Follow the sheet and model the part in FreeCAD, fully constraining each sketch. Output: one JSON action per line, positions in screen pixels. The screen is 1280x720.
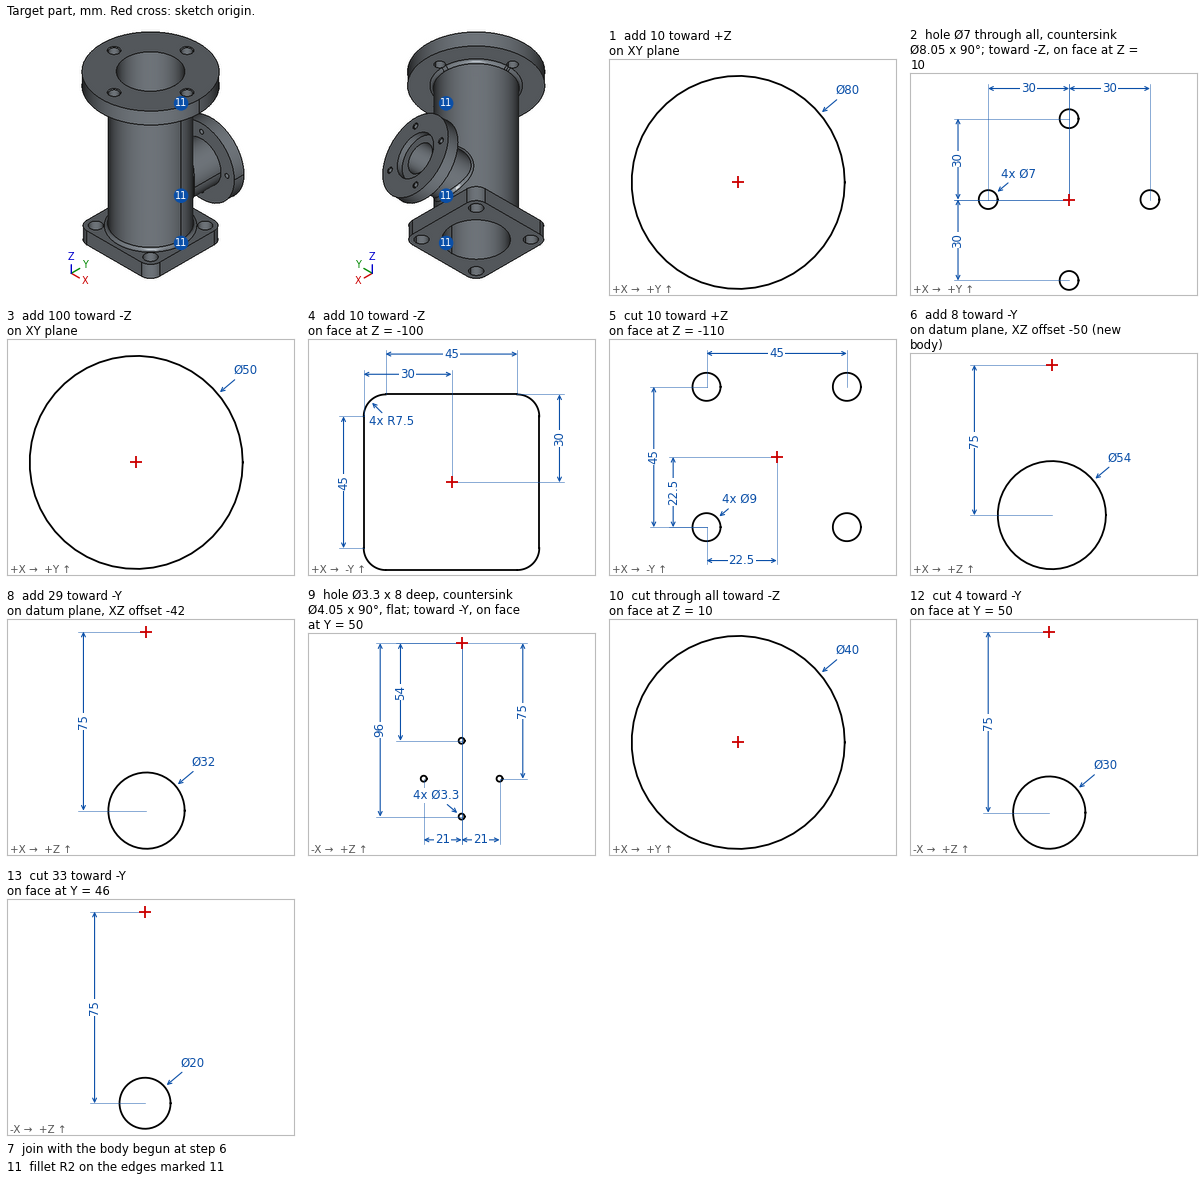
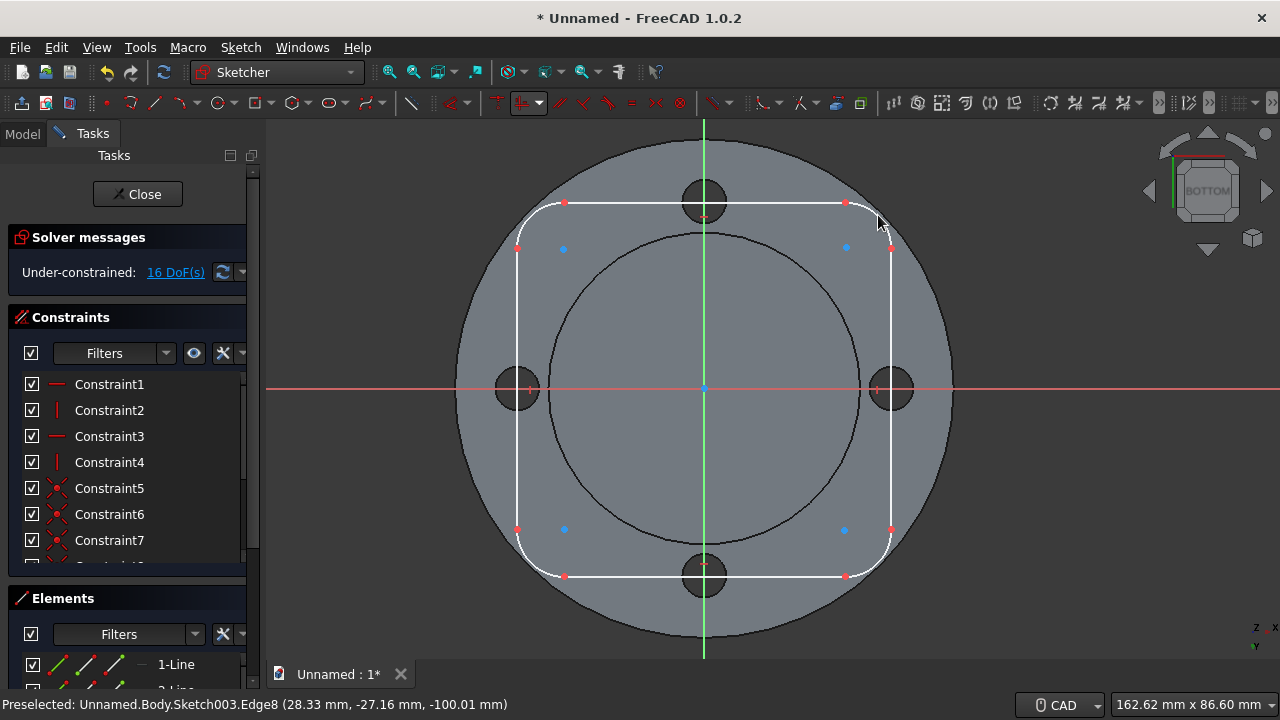
{"action": "left_click", "coordinate": [761, 203]}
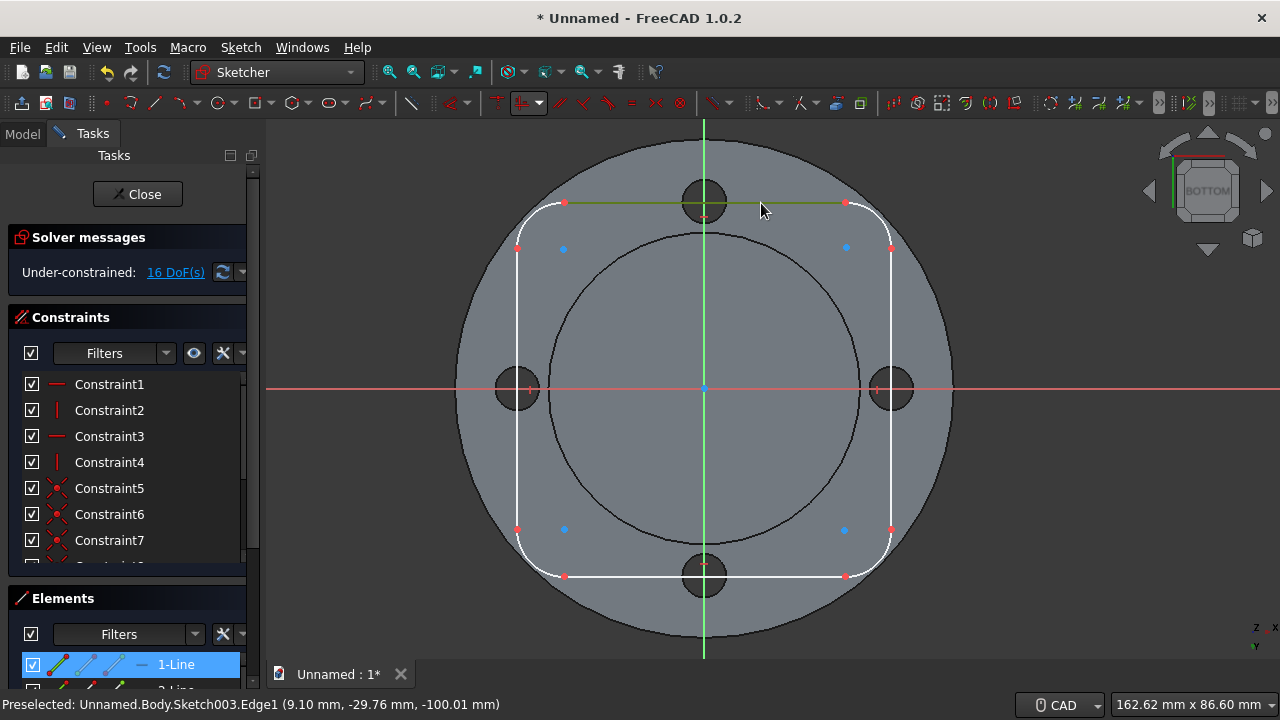
{"action": "left_click", "coordinate": [543, 208]}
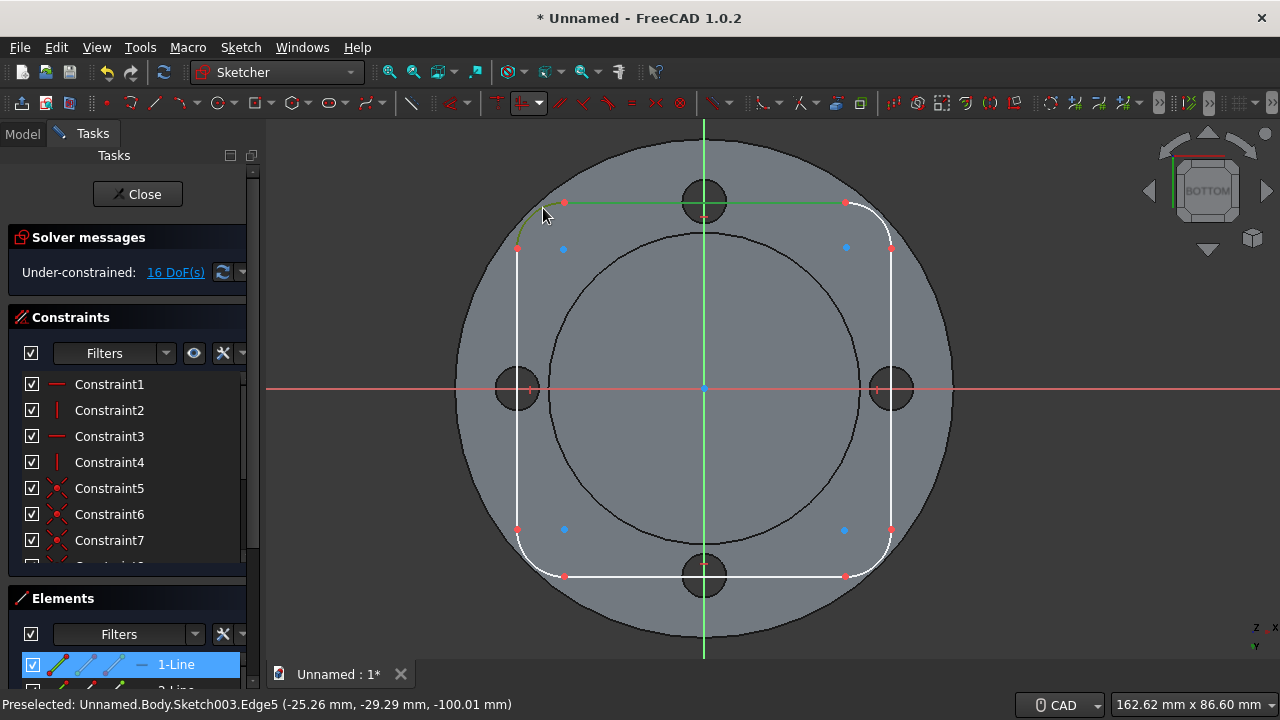
{"action": "left_click", "coordinate": [608, 104]}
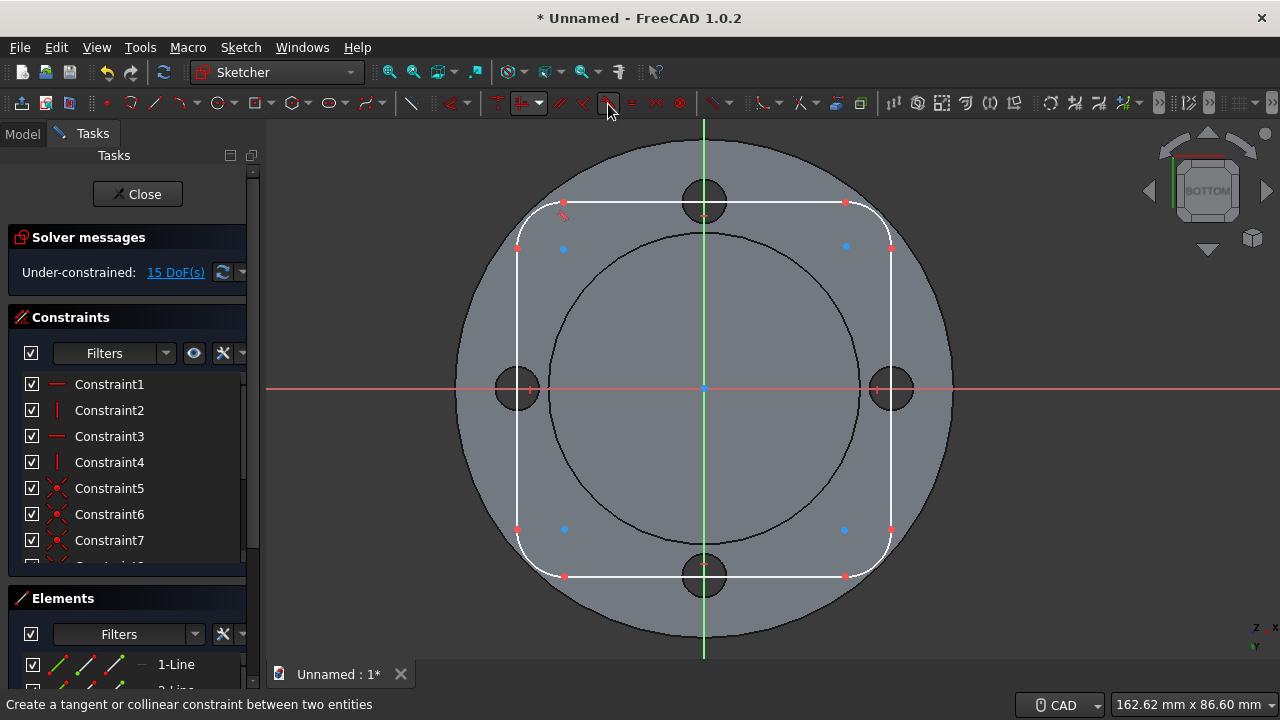
{"action": "left_click", "coordinate": [761, 202]}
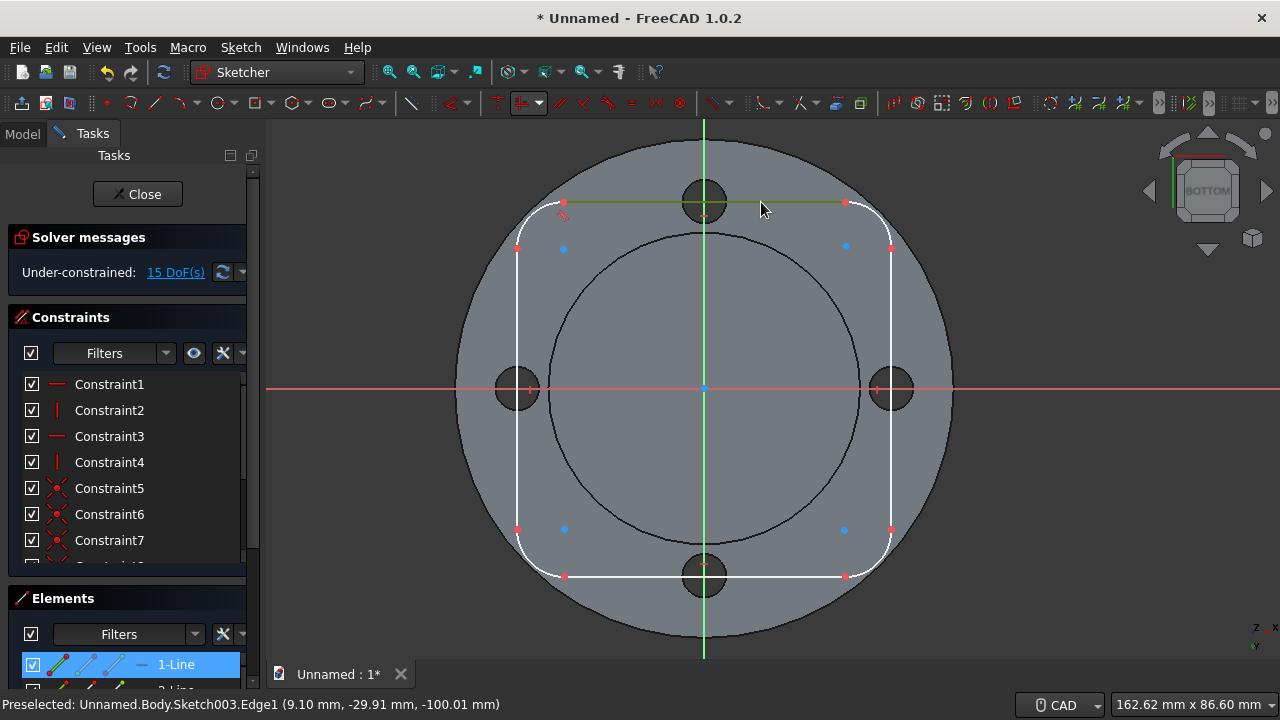
{"action": "left_click", "coordinate": [887, 228]}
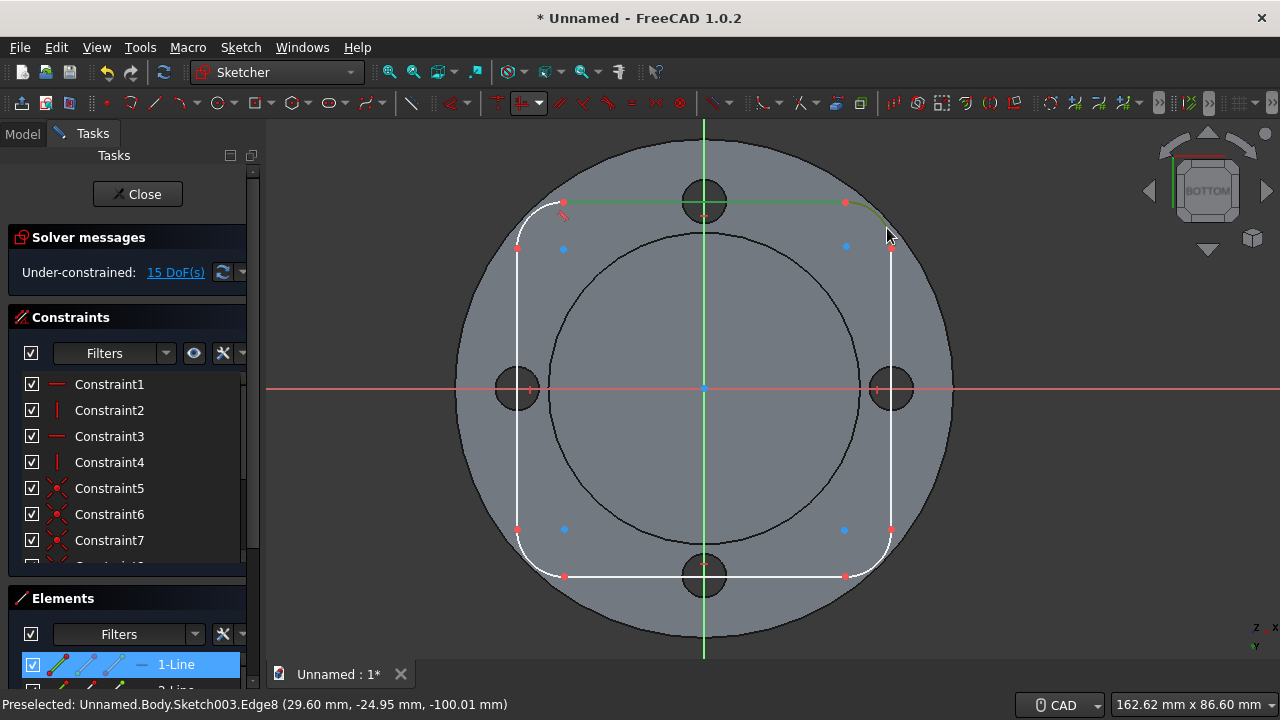
{"action": "left_click", "coordinate": [608, 104]}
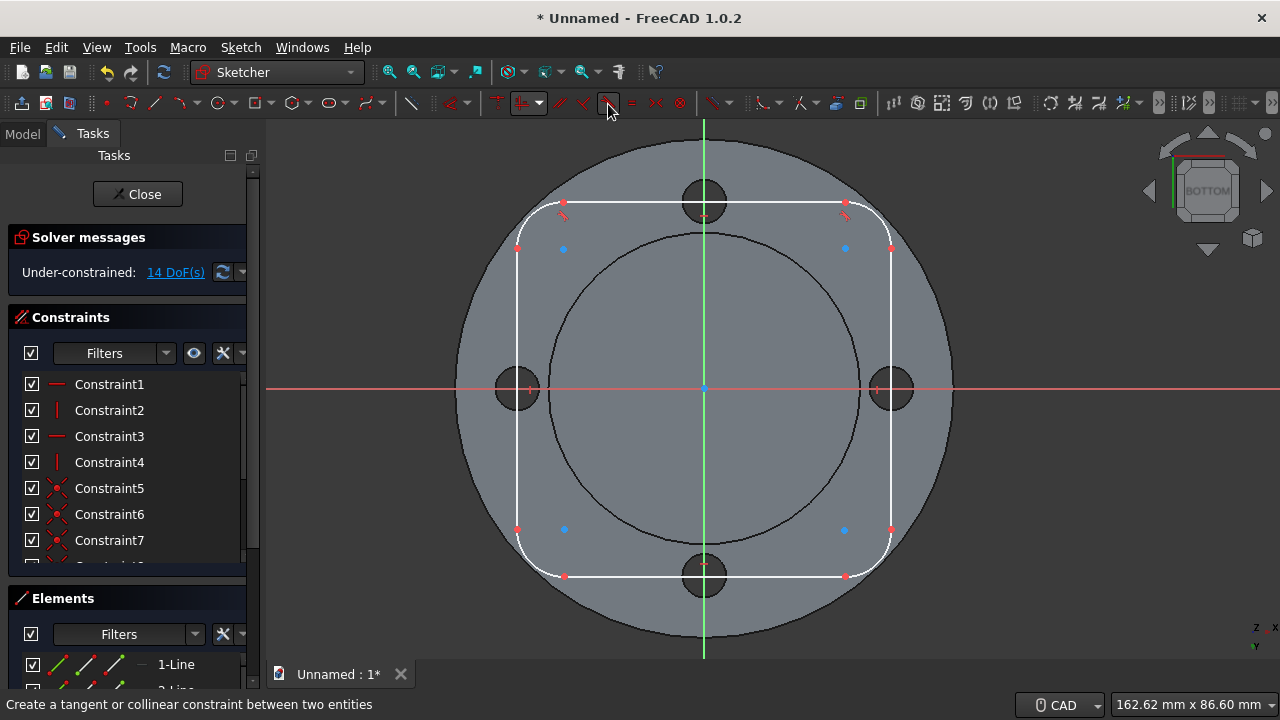
{"action": "left_click", "coordinate": [517, 333]}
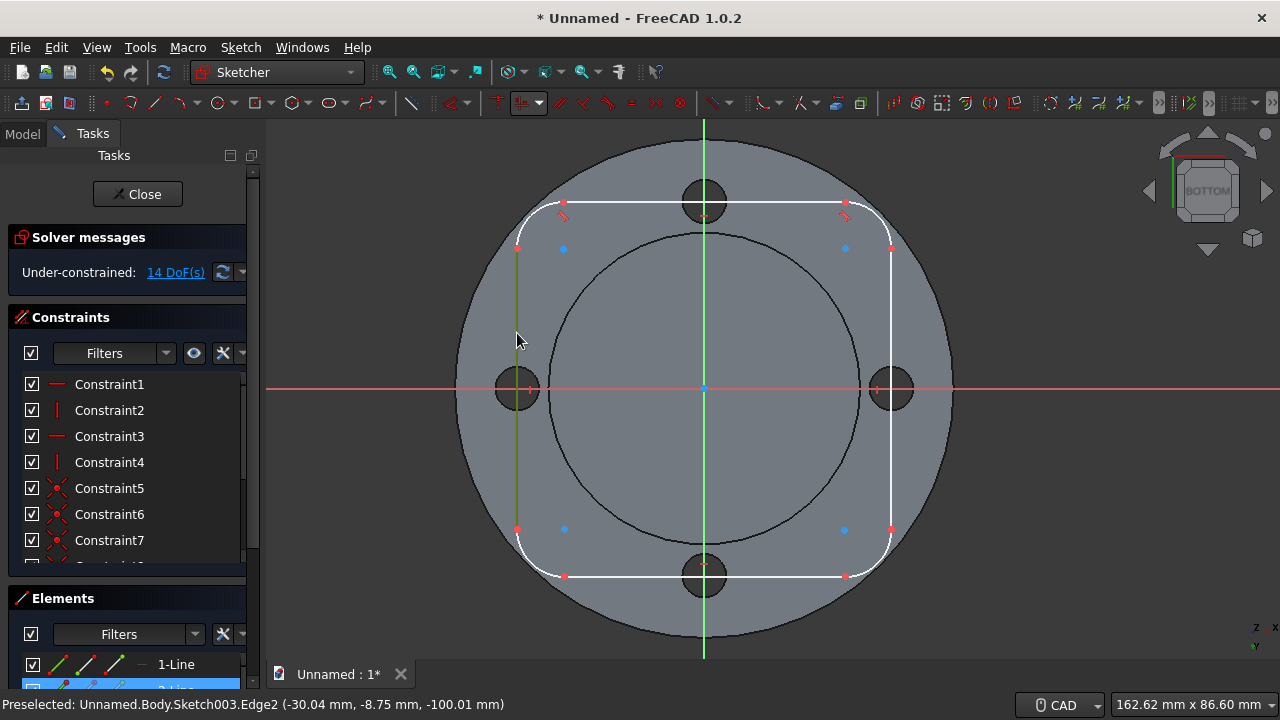
{"action": "left_click", "coordinate": [543, 207]}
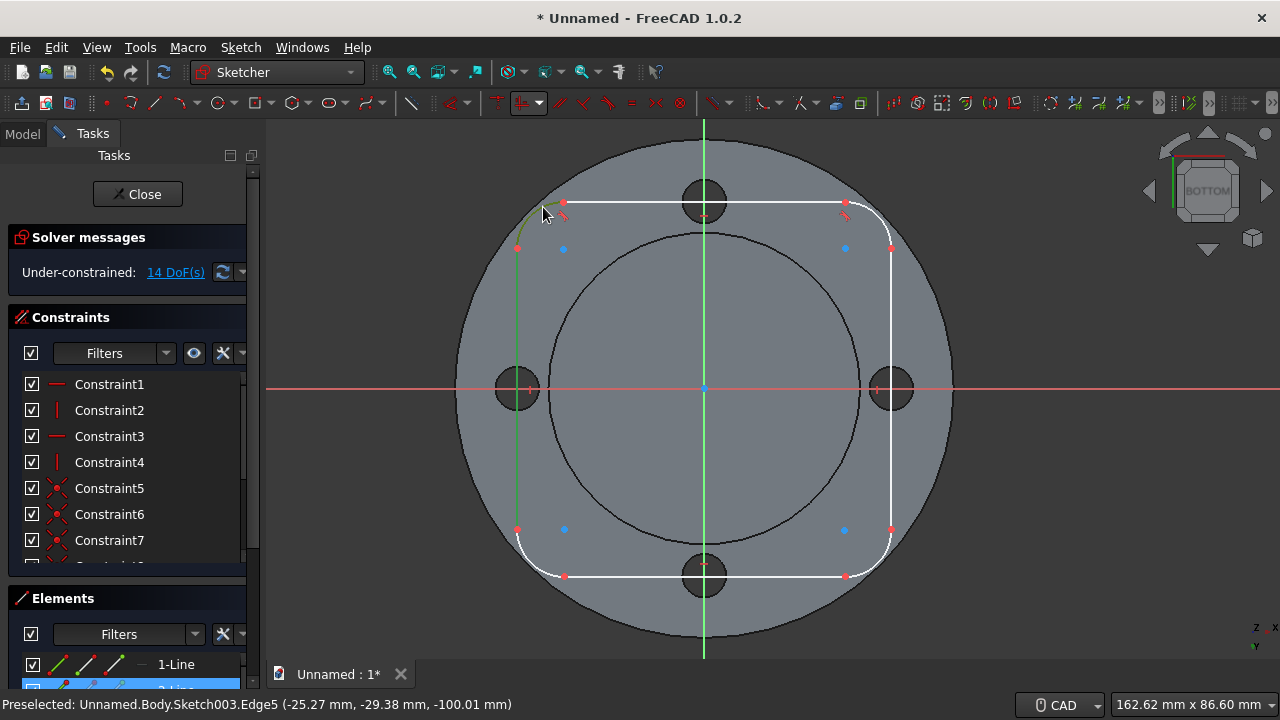
{"action": "left_click", "coordinate": [608, 104]}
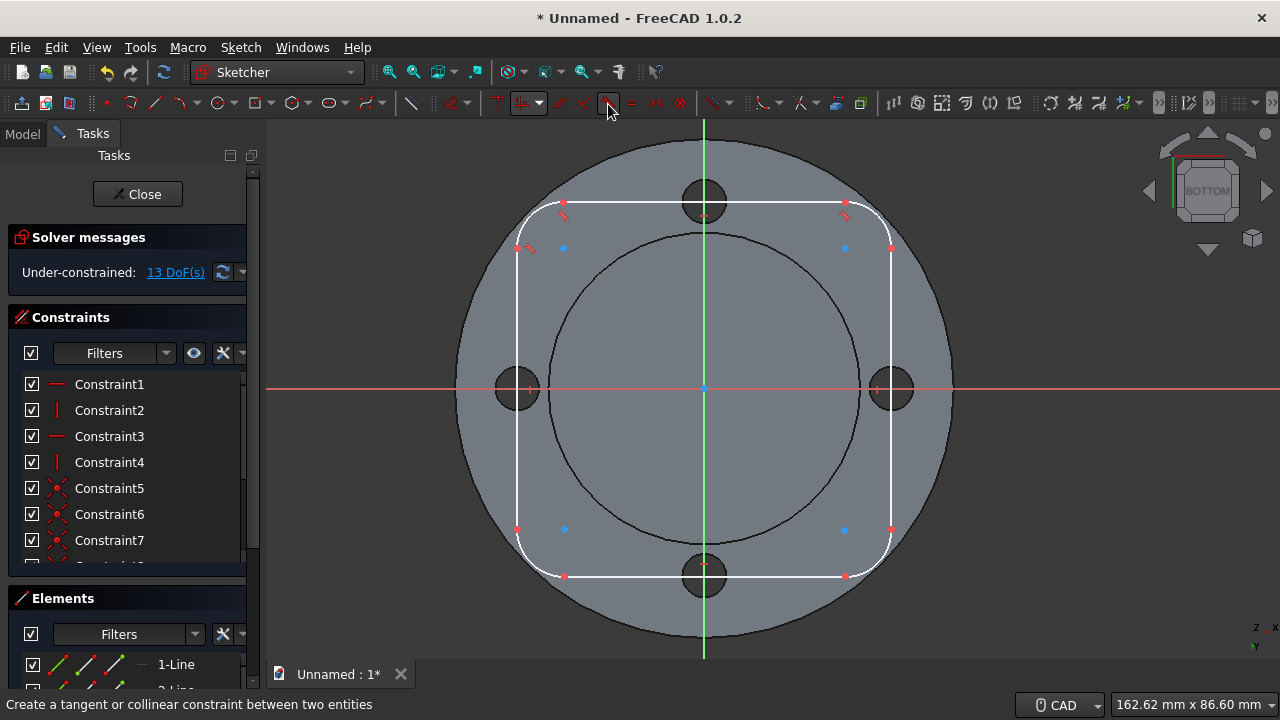
{"action": "left_click", "coordinate": [517, 333]}